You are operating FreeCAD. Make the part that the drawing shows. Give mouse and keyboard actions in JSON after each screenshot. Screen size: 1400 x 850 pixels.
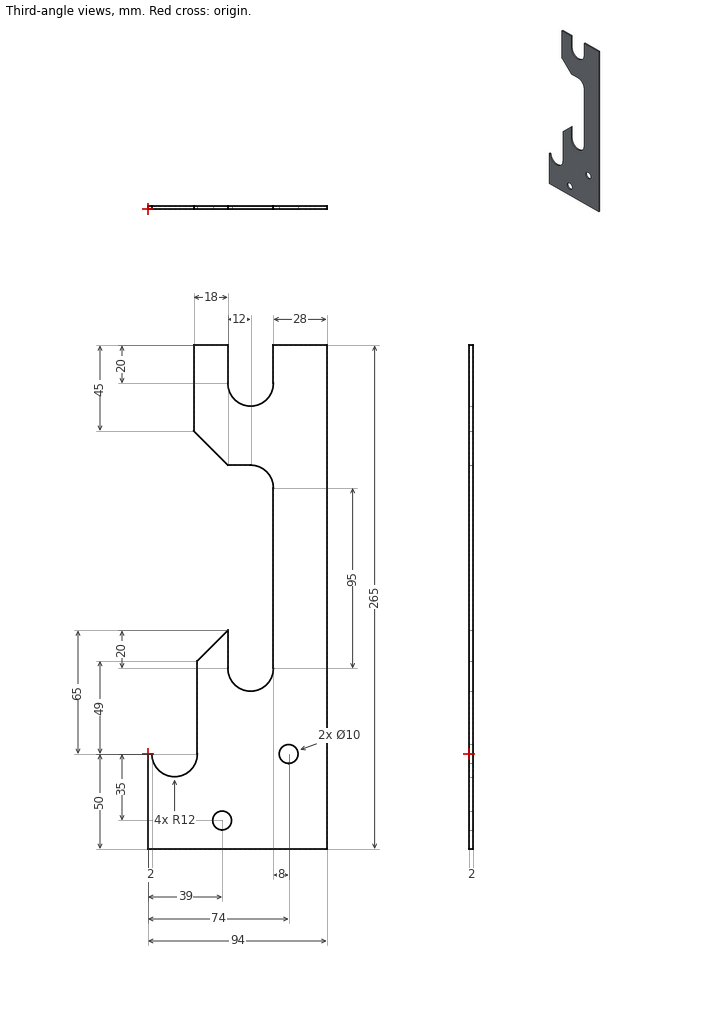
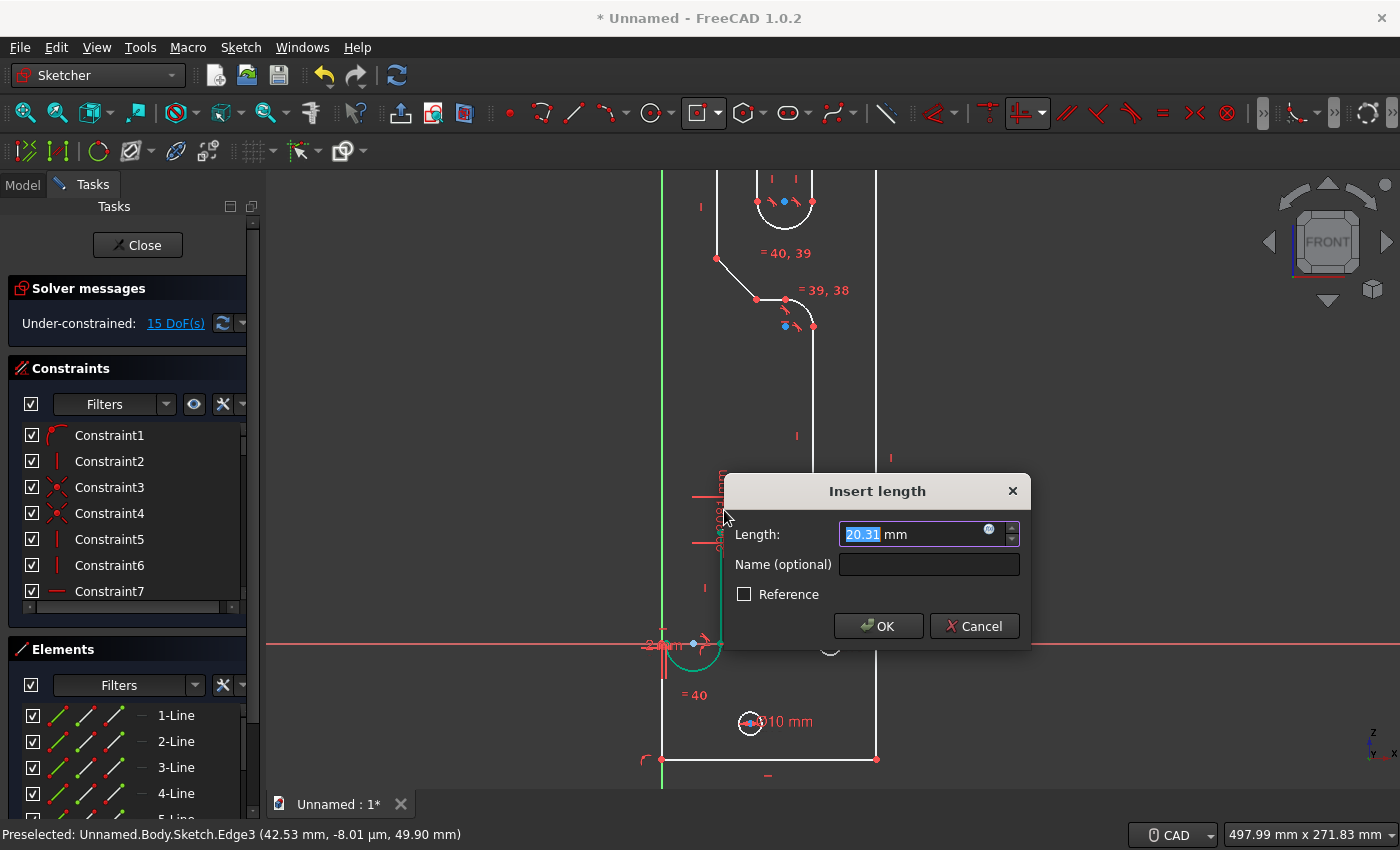
{"action": "type", "text": "20"}
{"action": "key", "text": "Return"}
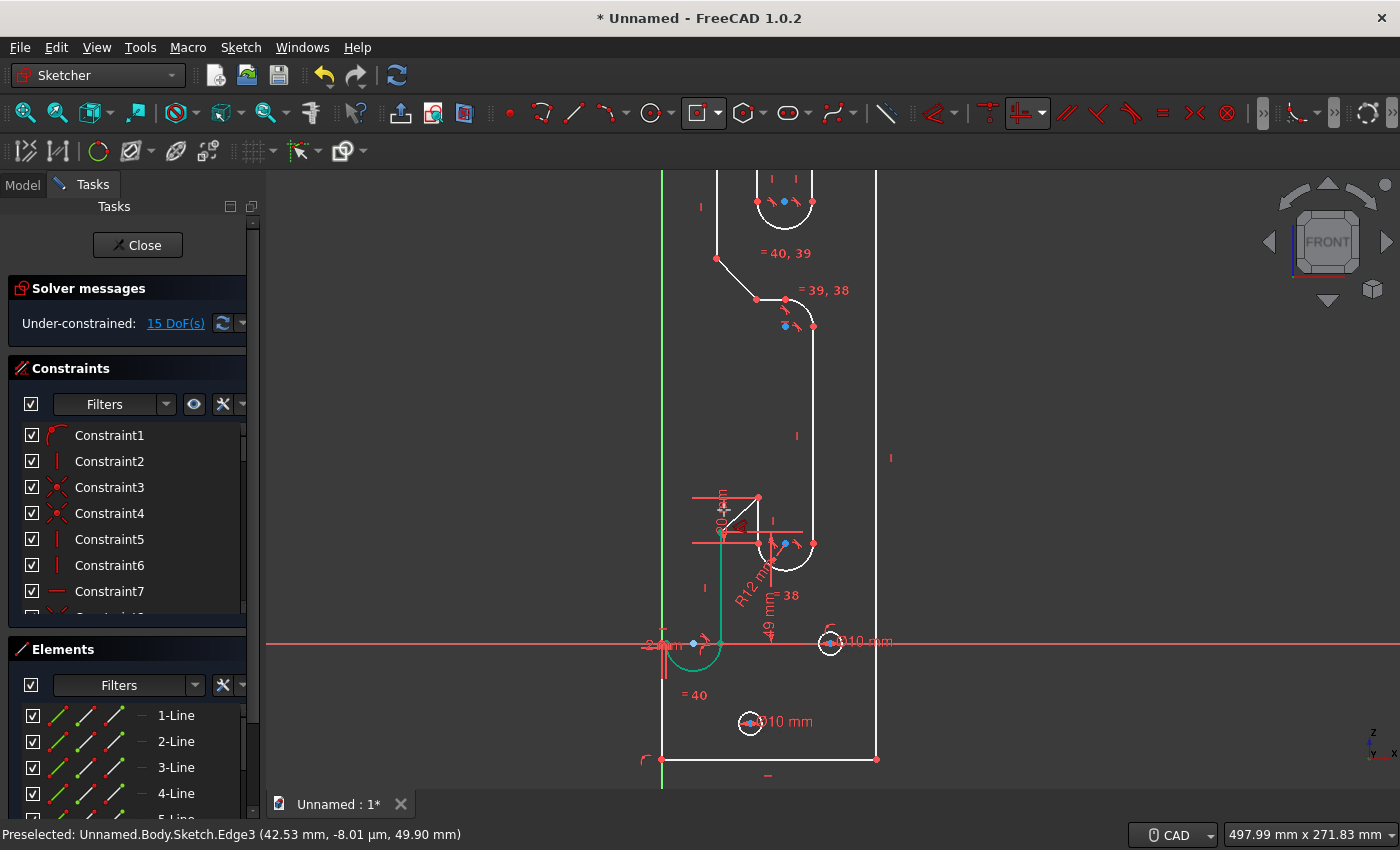
{"action": "left_click", "coordinate": [813, 478]}
{"action": "left_click", "coordinate": [847, 435]}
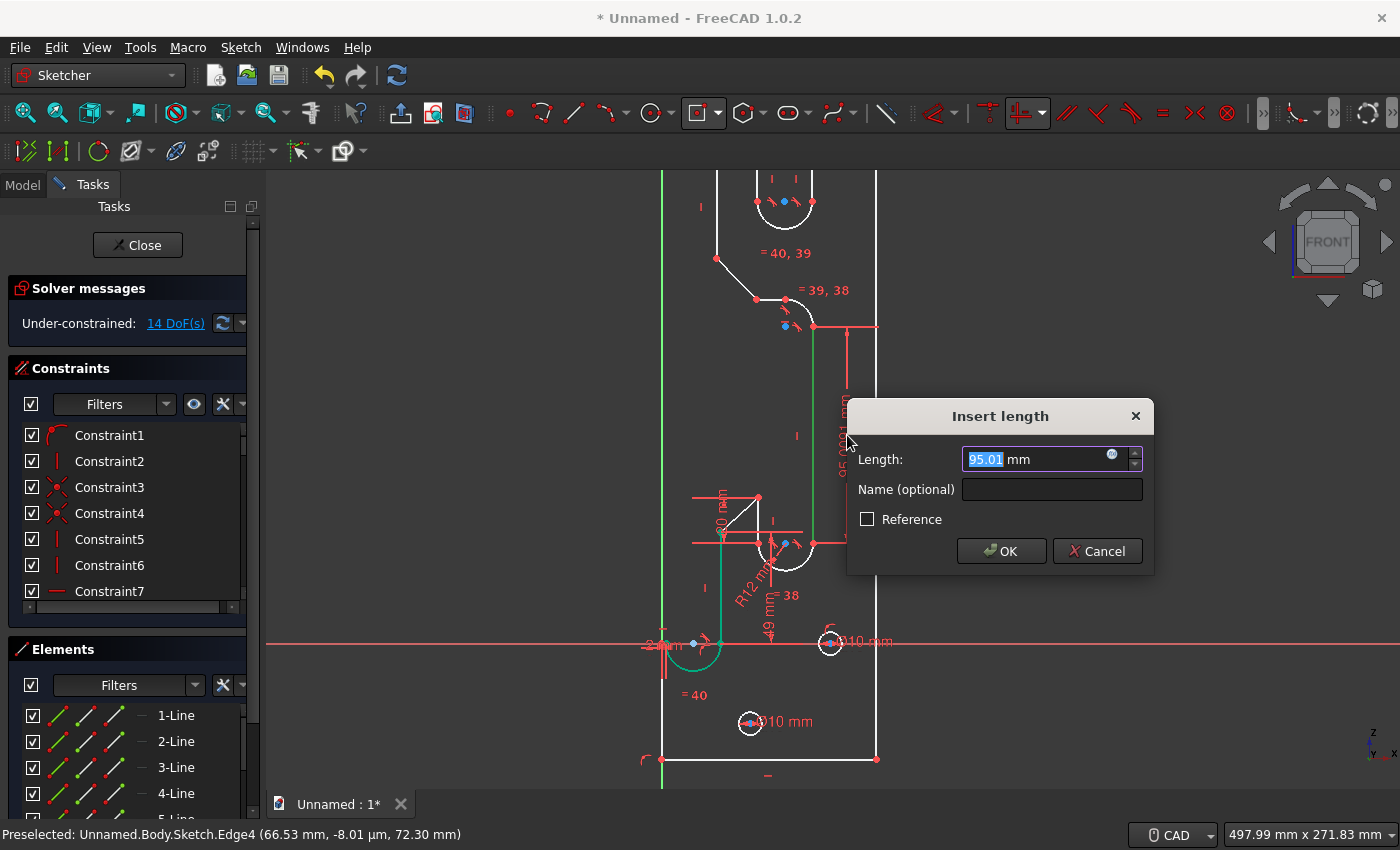
{"action": "type", "text": "95"}
{"action": "key", "text": "Return"}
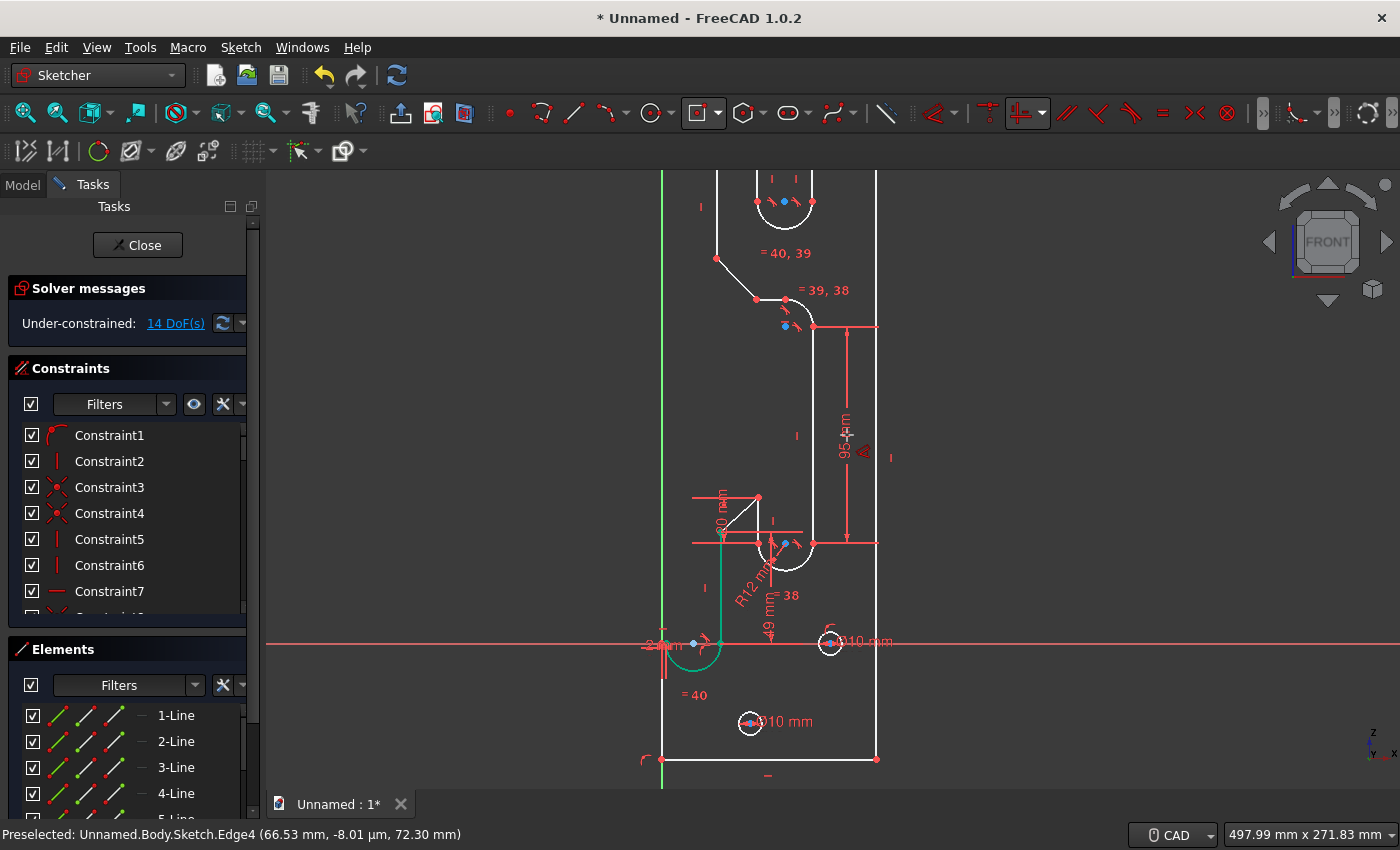
{"action": "scroll", "coordinate": [774, 300], "scroll_direction": "up", "scroll_amount": 2}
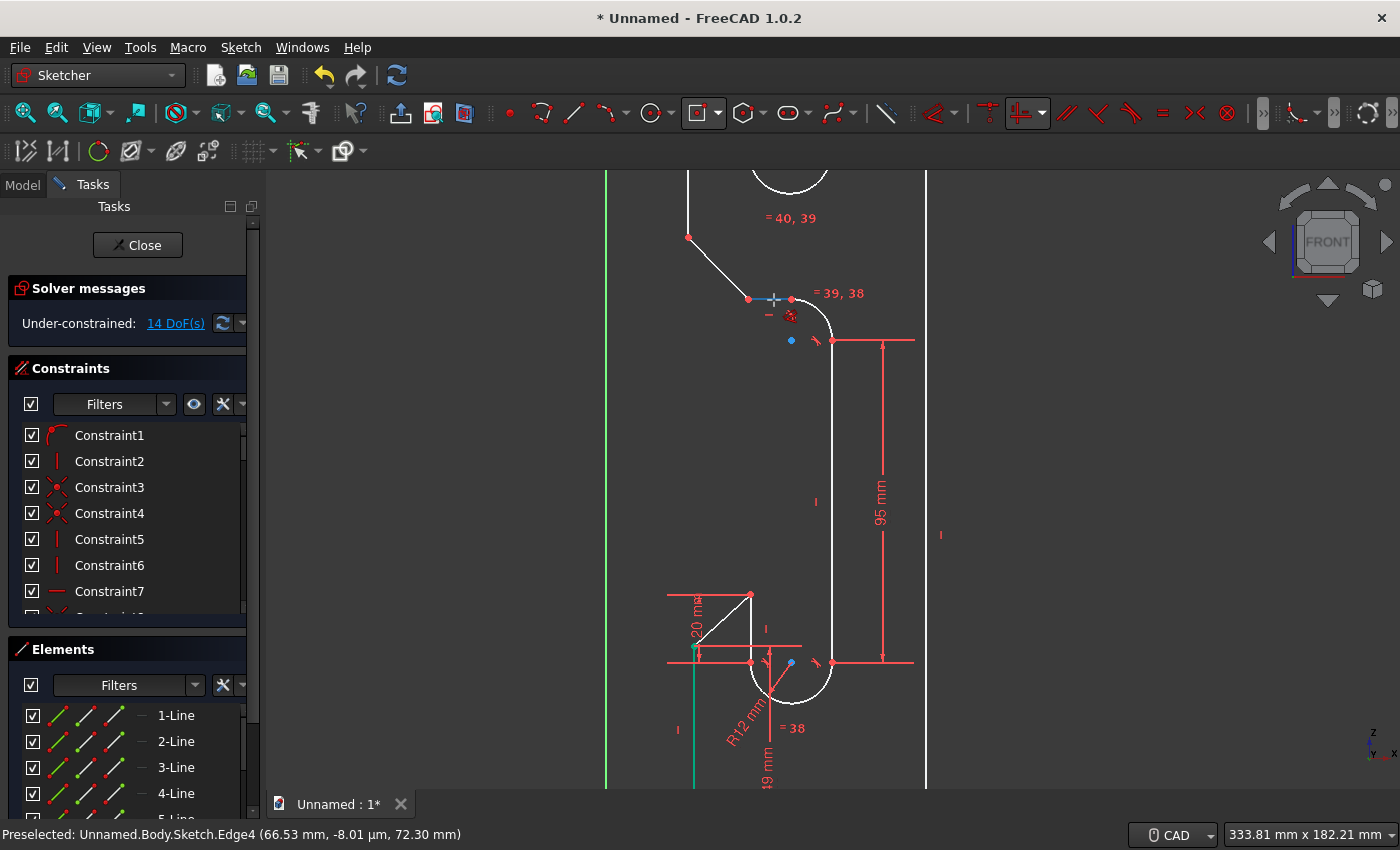
{"action": "left_click", "coordinate": [774, 299]}
{"action": "left_click", "coordinate": [770, 265]}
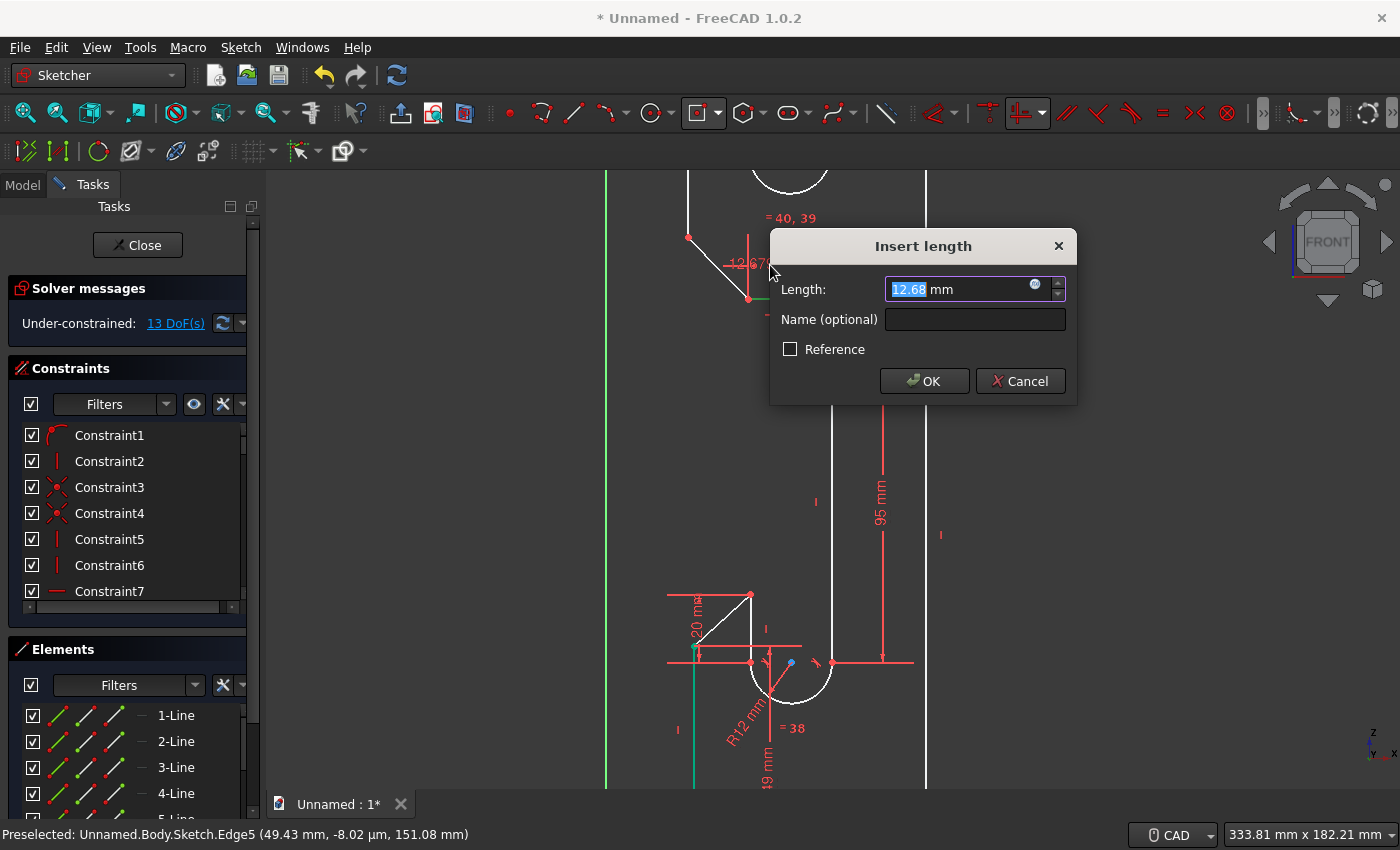
{"action": "type", "text": "12"}
{"action": "key", "text": "Return"}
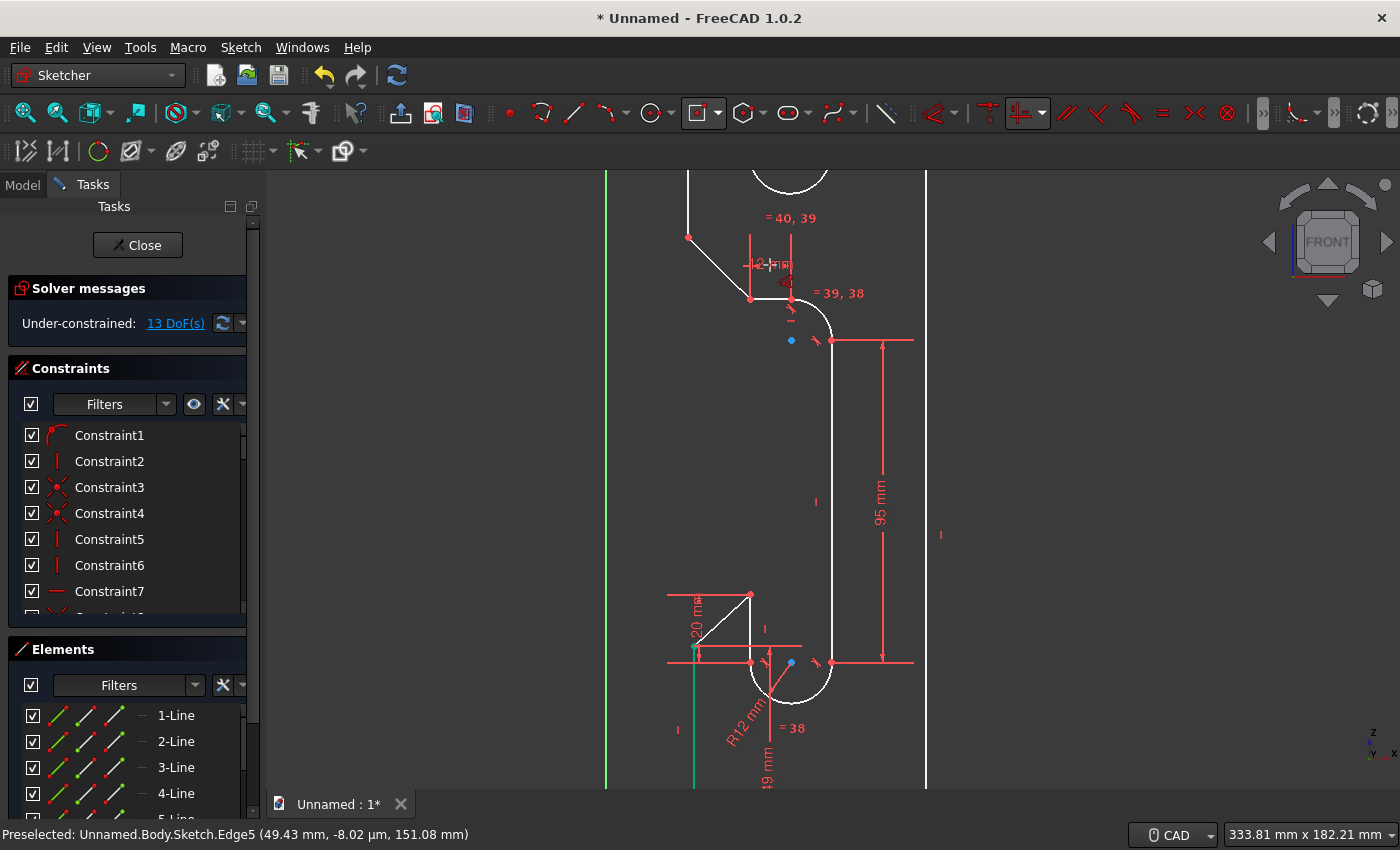
{"action": "left_click", "coordinate": [688, 207]}
{"action": "left_click", "coordinate": [654, 218]}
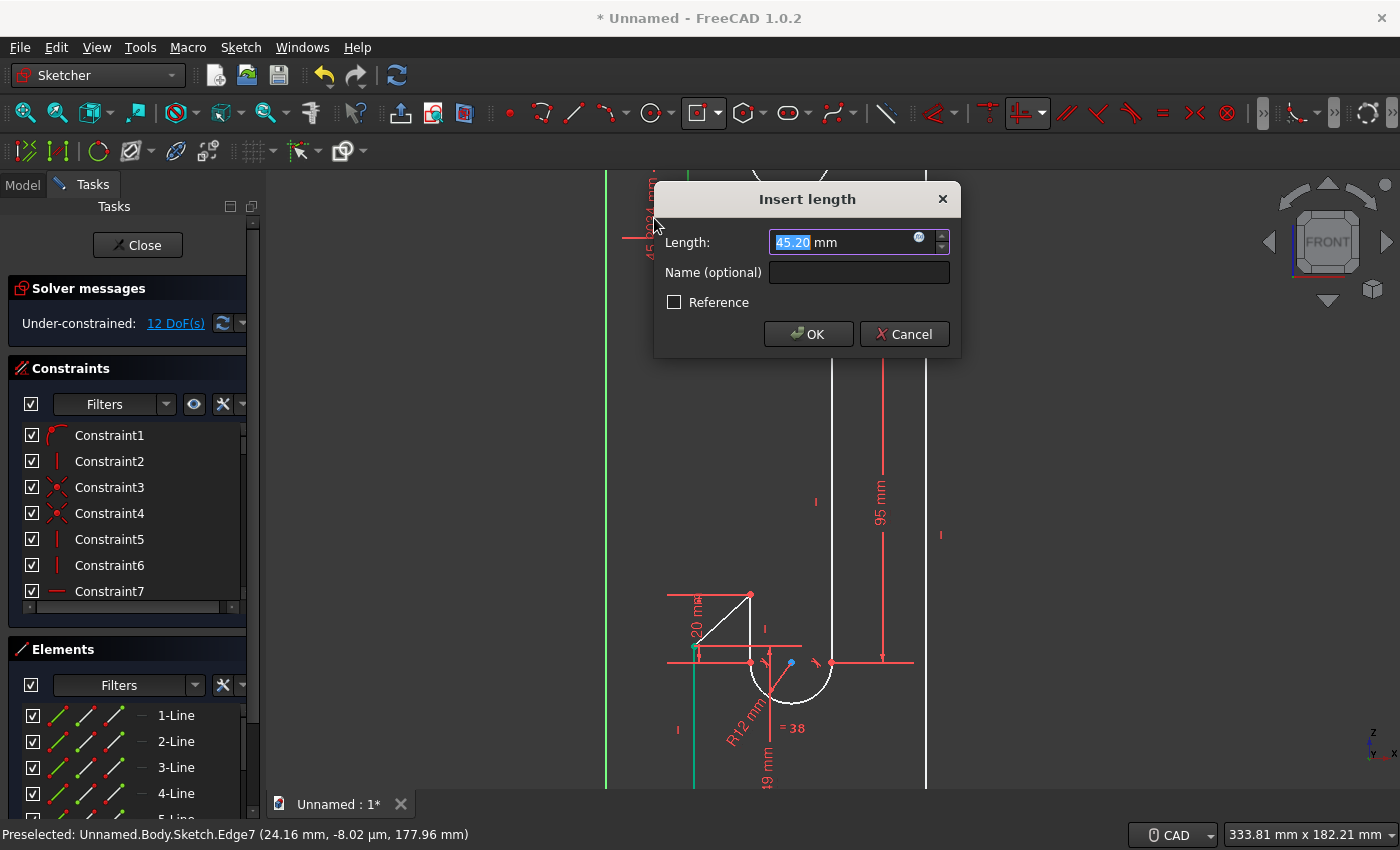
{"action": "type", "text": "45"}
{"action": "key", "text": "Return"}